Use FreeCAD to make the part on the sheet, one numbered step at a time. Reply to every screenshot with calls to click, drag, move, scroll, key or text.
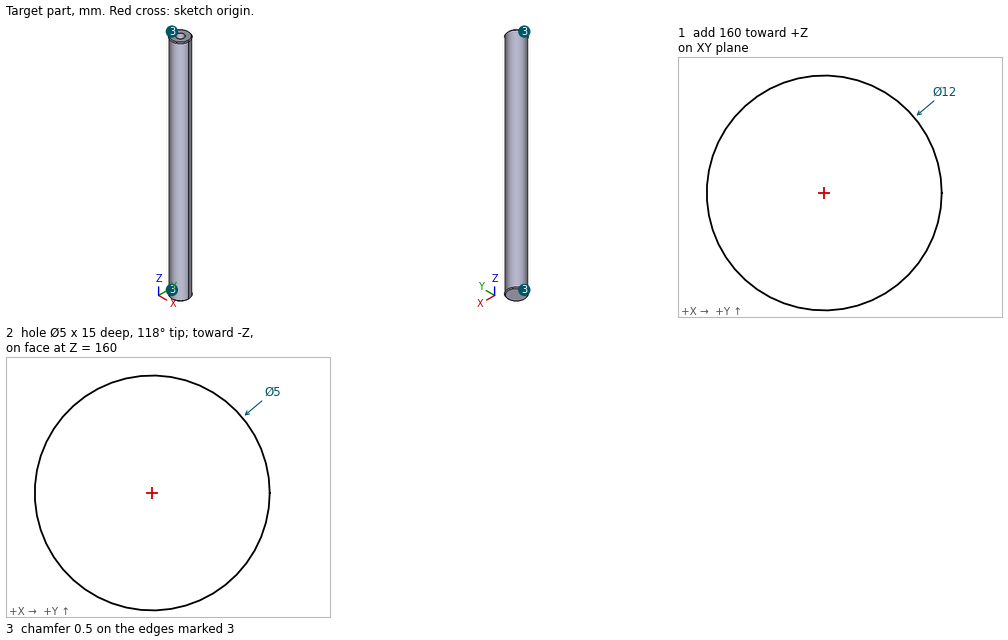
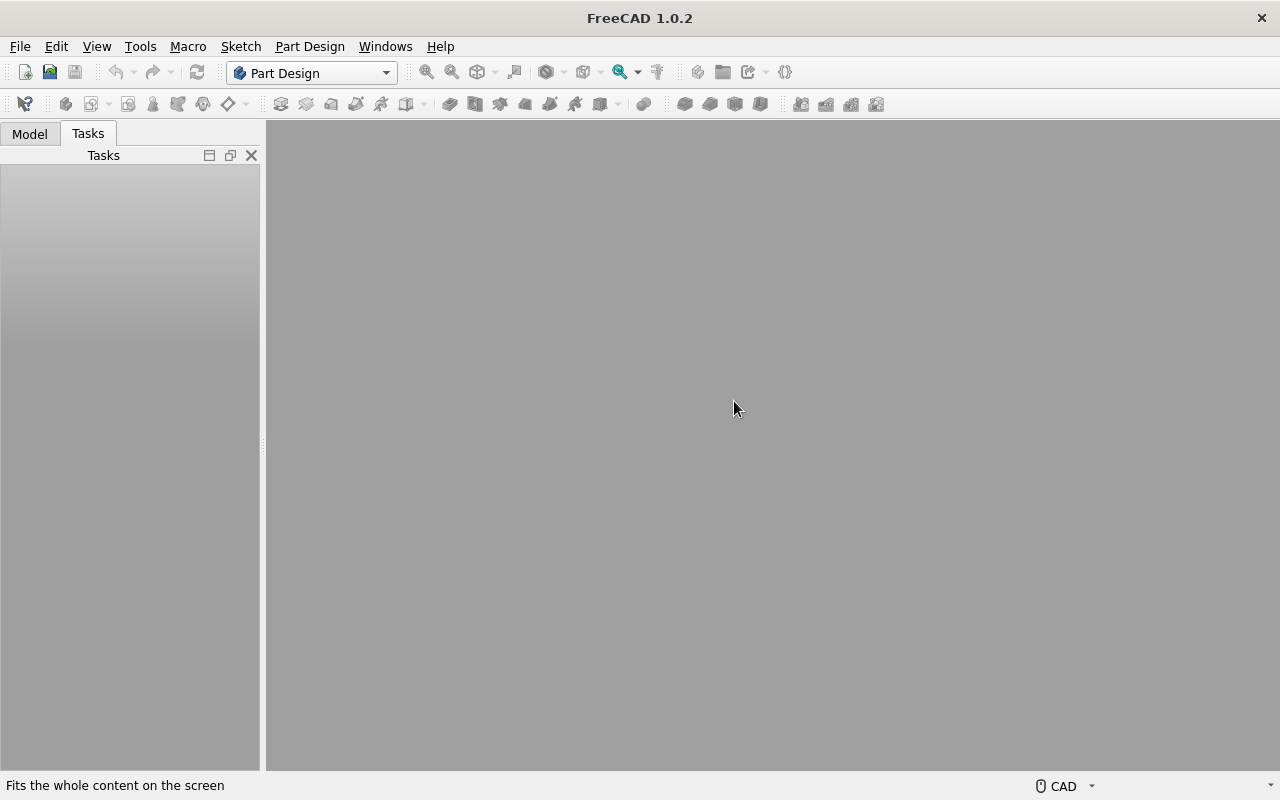
click(25, 72)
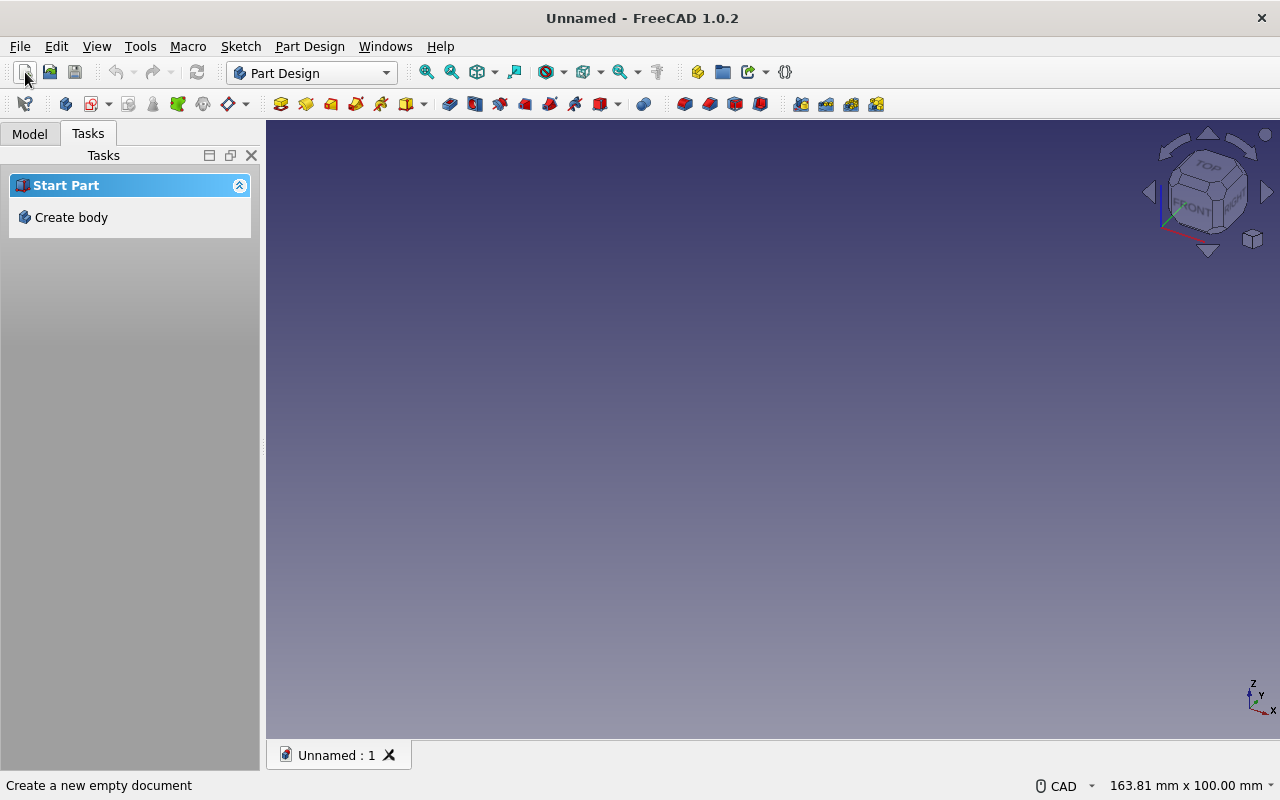
click(90, 104)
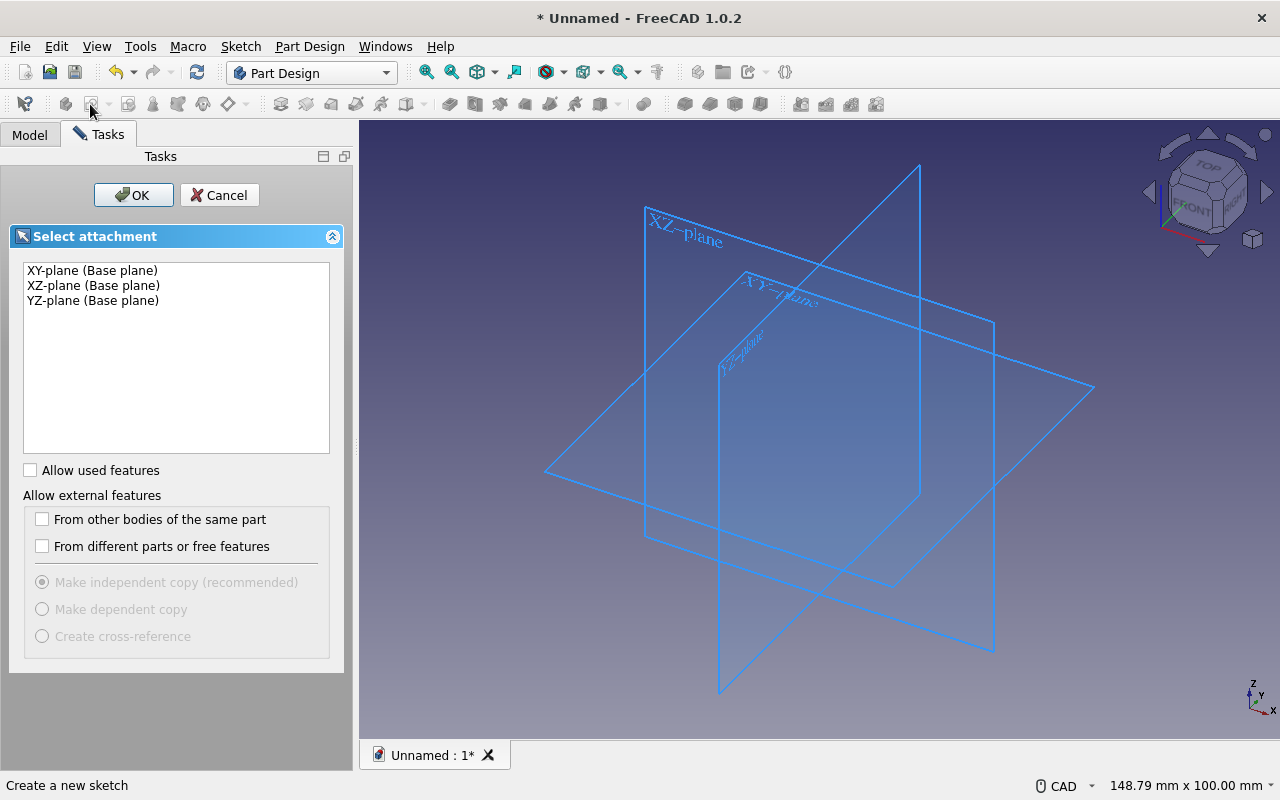
click(84, 270)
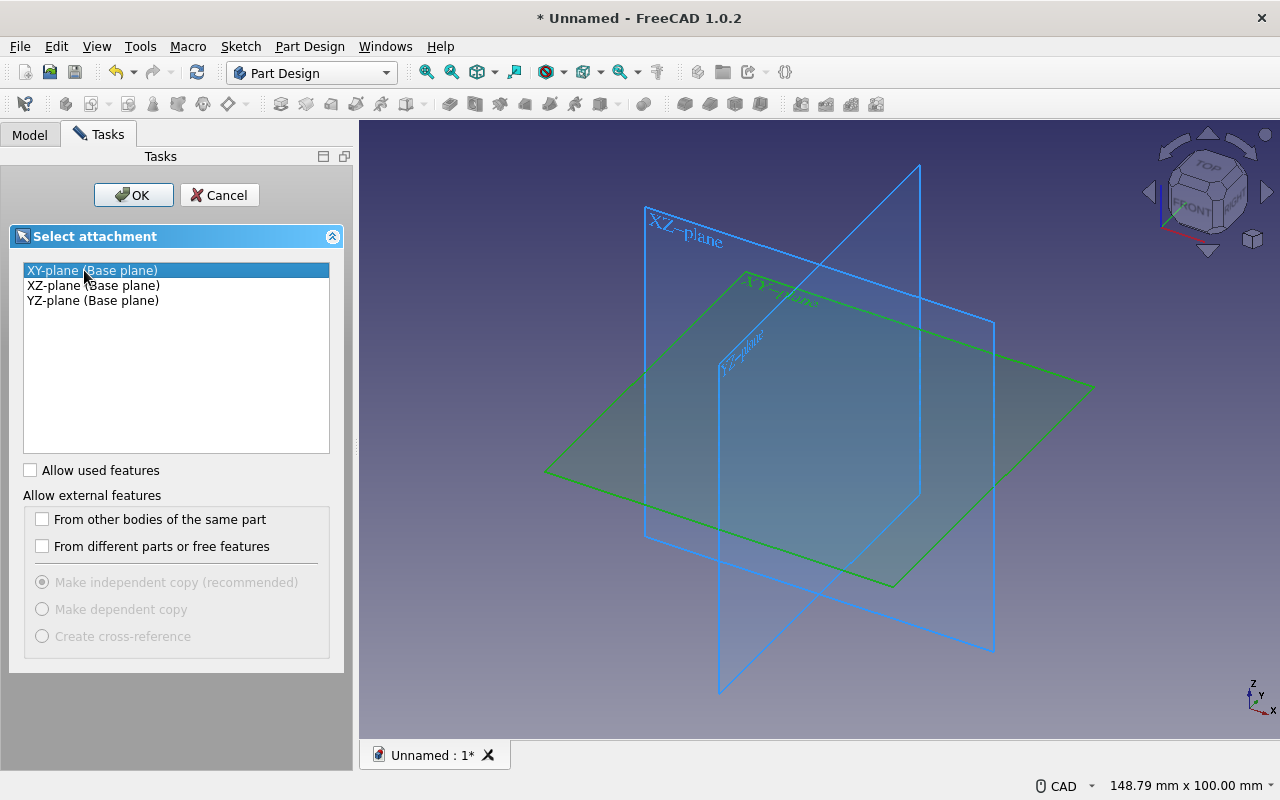
click(134, 195)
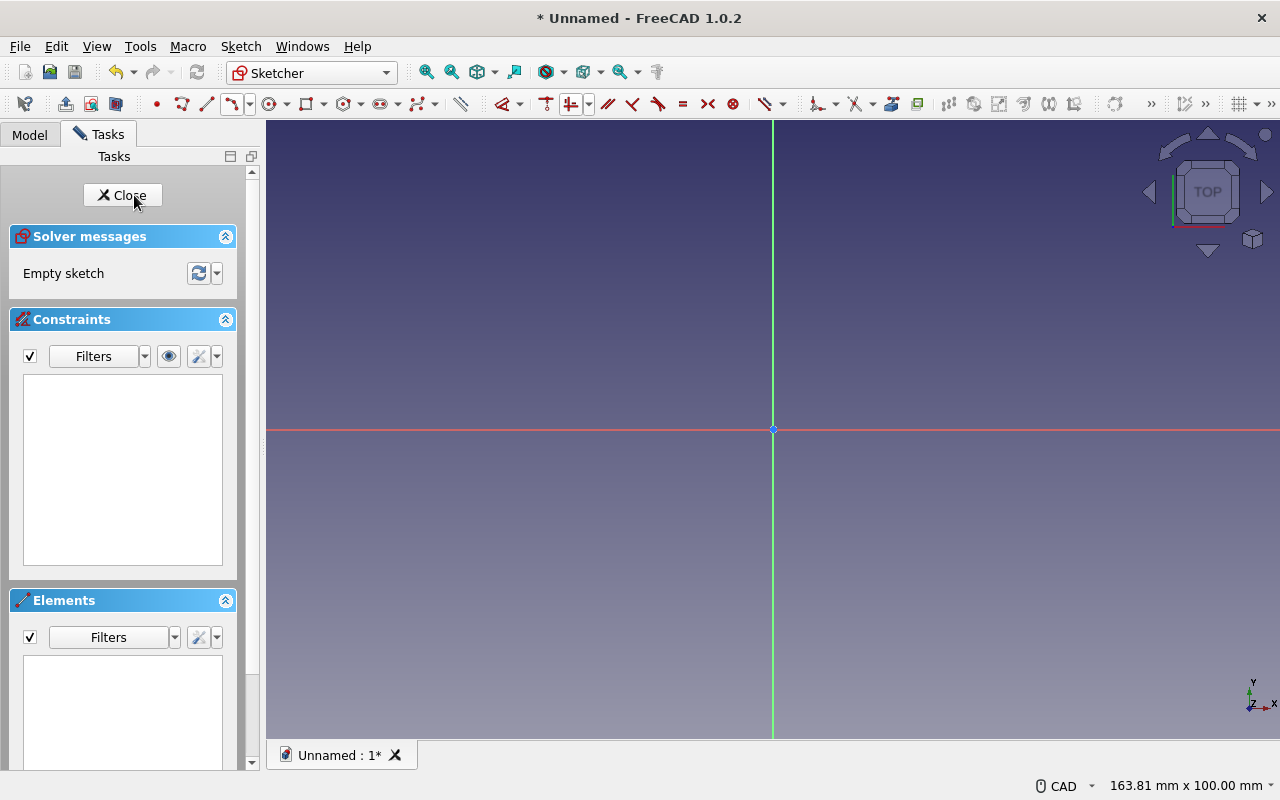
scroll(790, 430, up, 8)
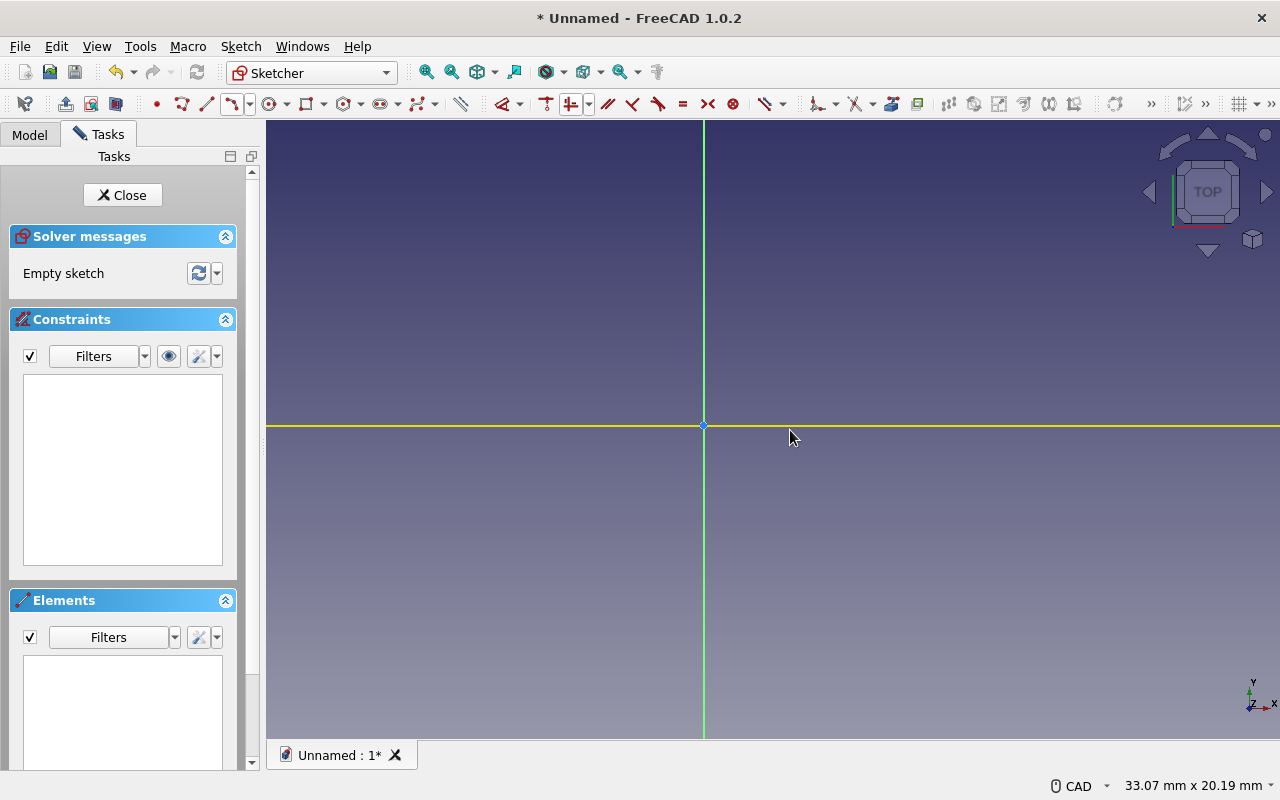
click(268, 104)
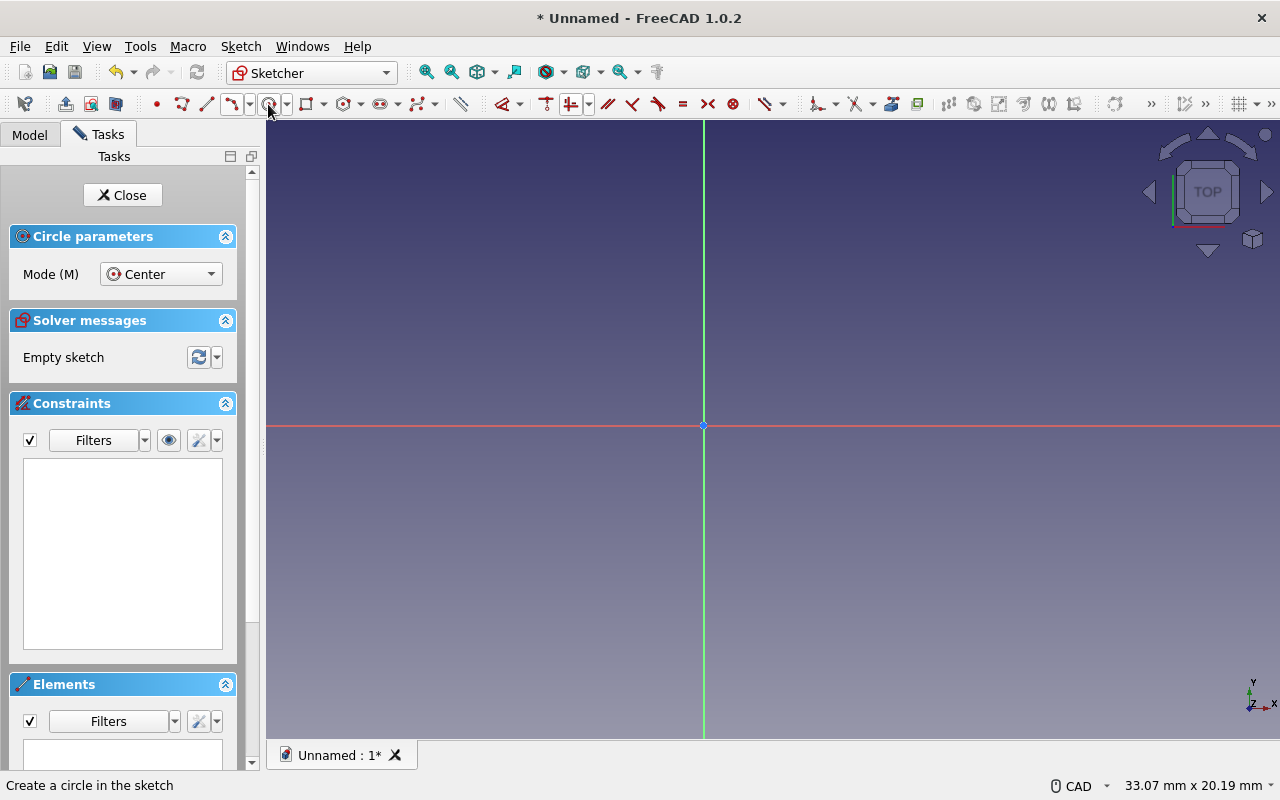
click(704, 426)
move(834, 295)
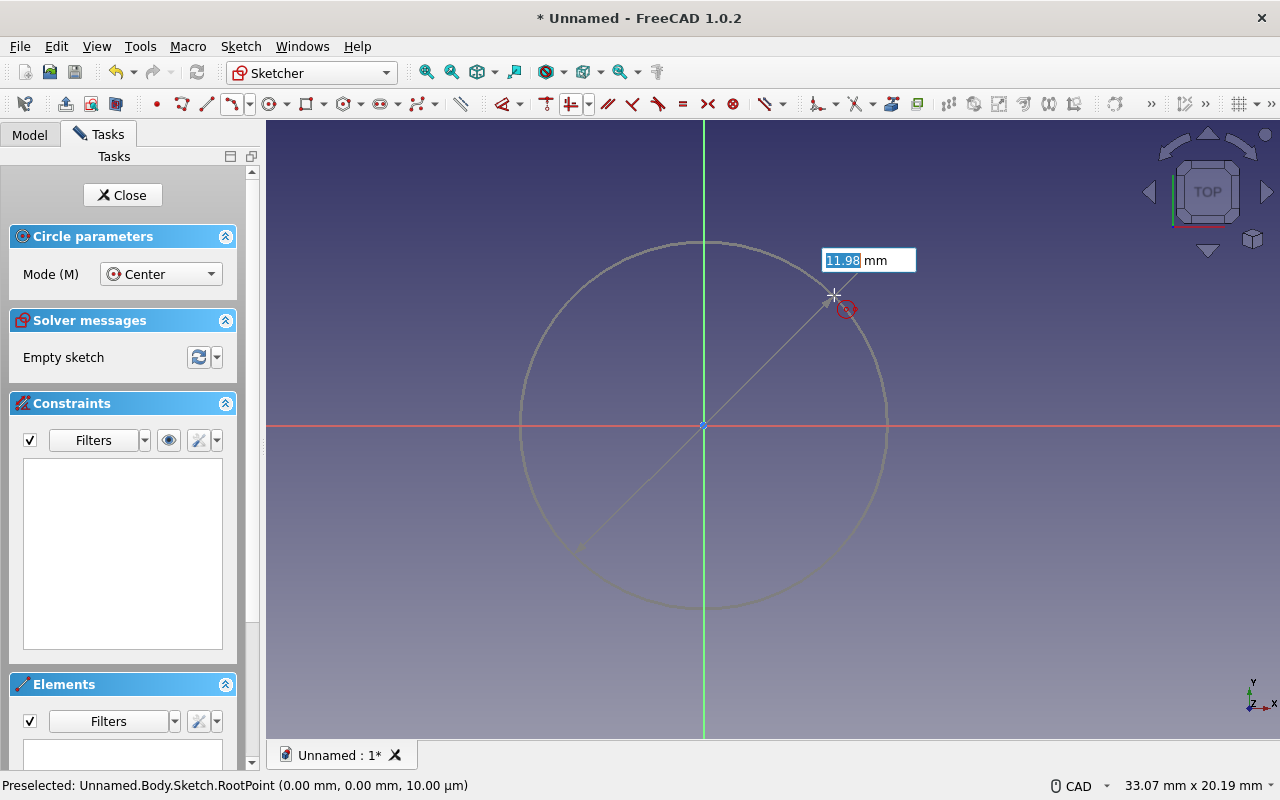
text(12)
key(Return)
key(Escape)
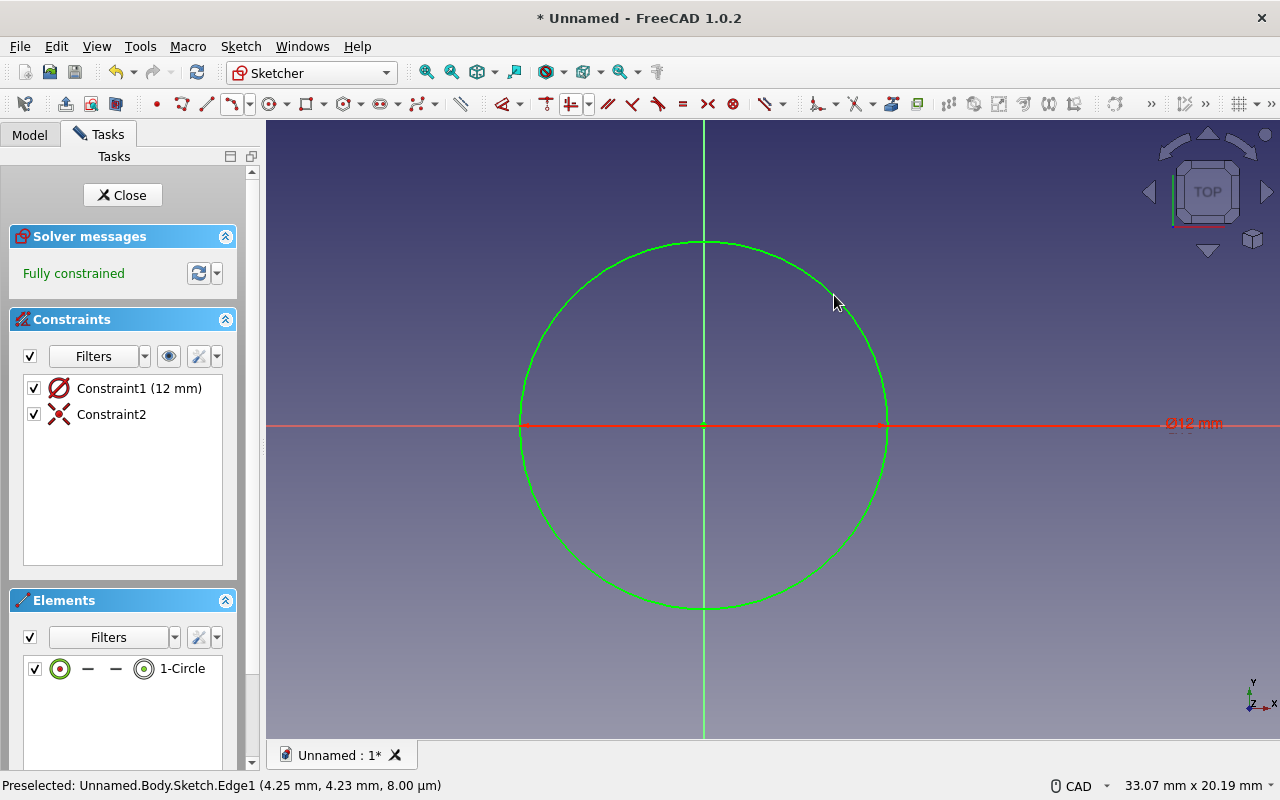
click(123, 195)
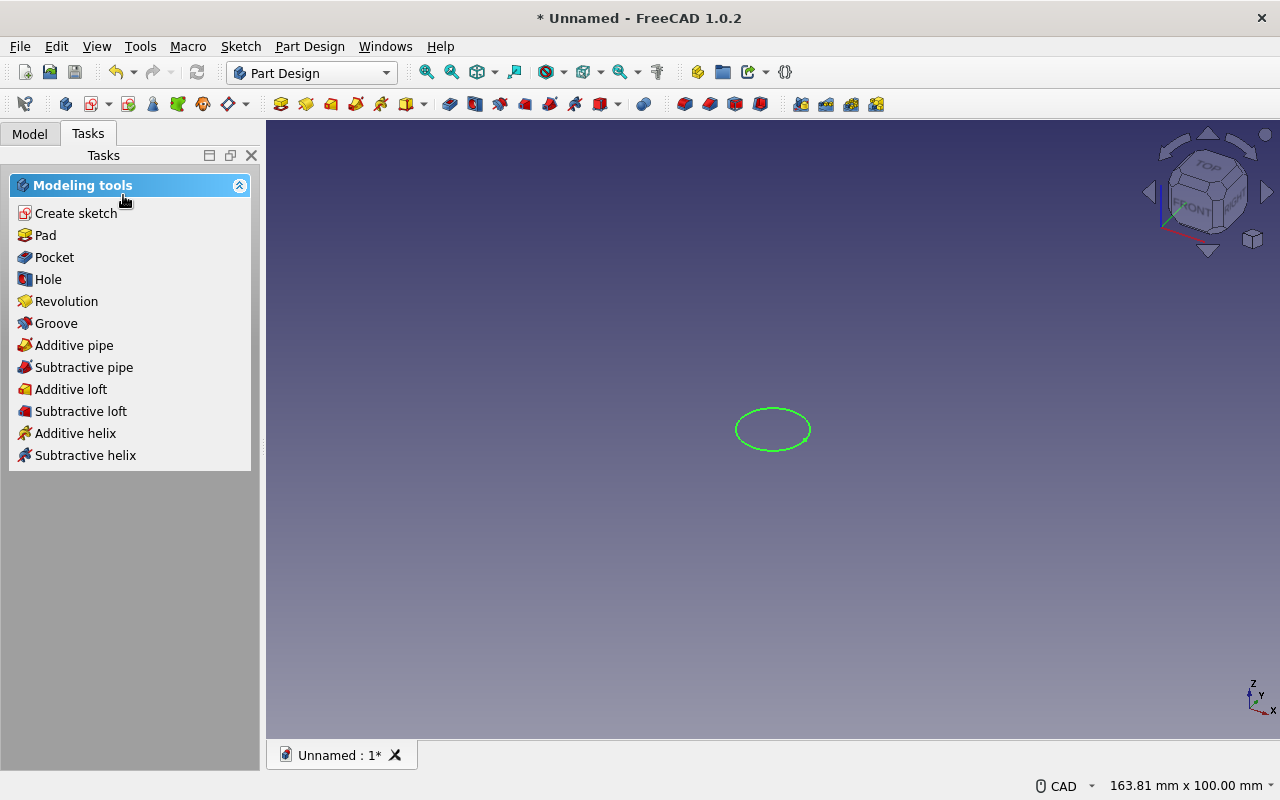
click(281, 104)